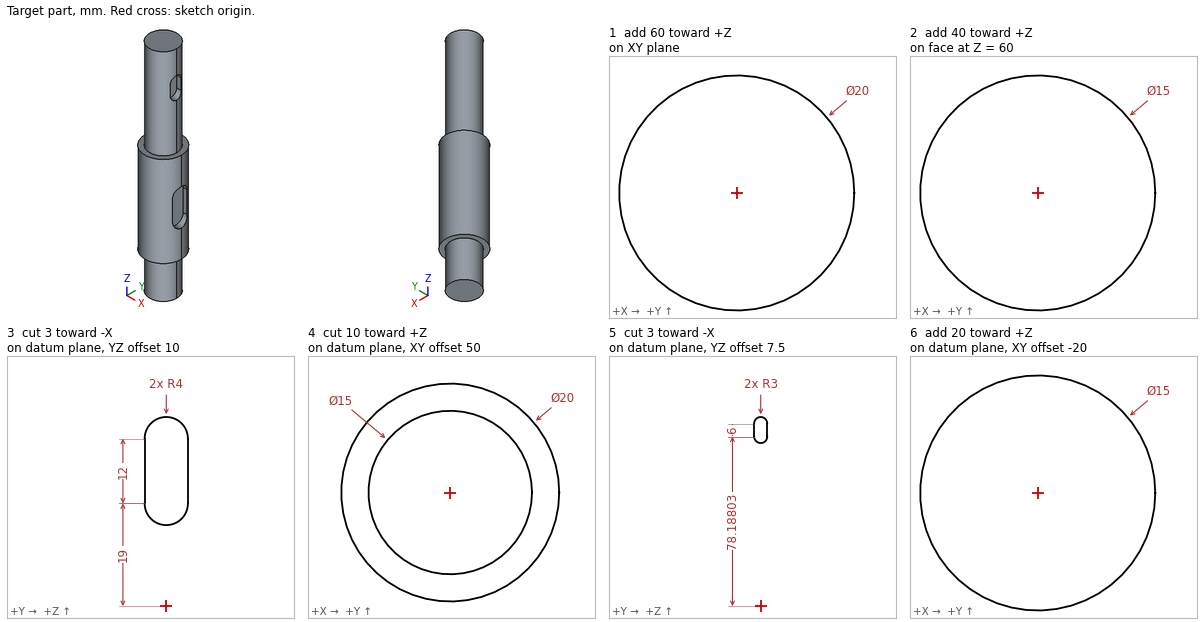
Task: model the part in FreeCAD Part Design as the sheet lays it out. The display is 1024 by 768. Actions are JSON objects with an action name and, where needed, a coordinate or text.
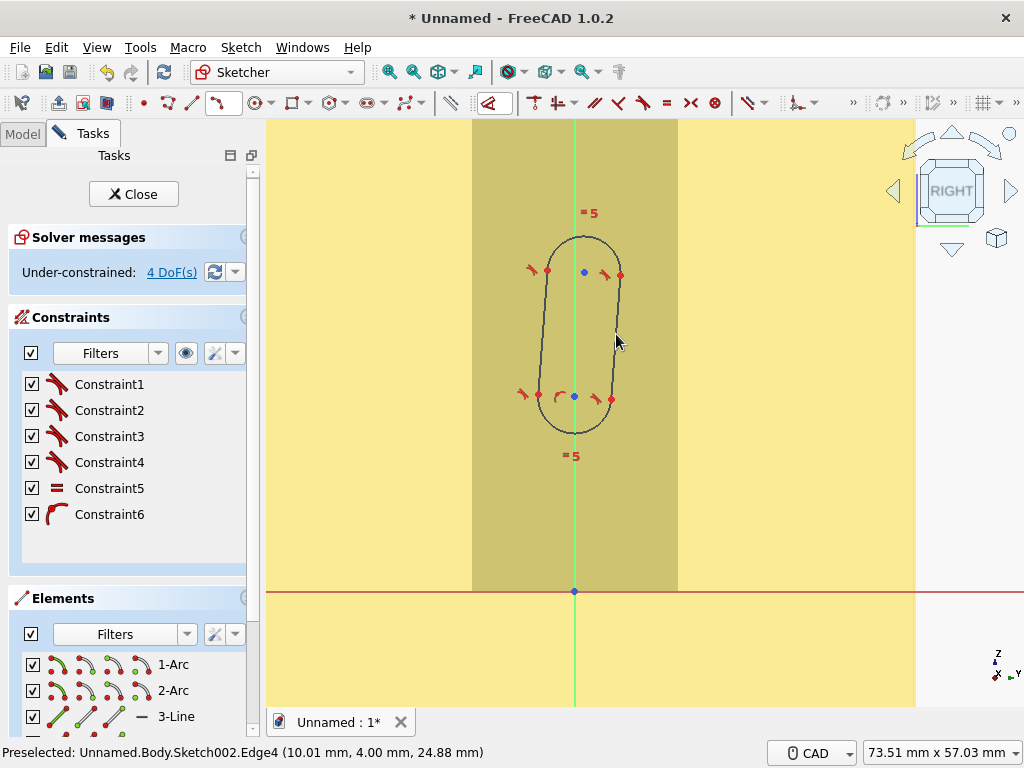
{"action": "left_click", "coordinate": [541, 357]}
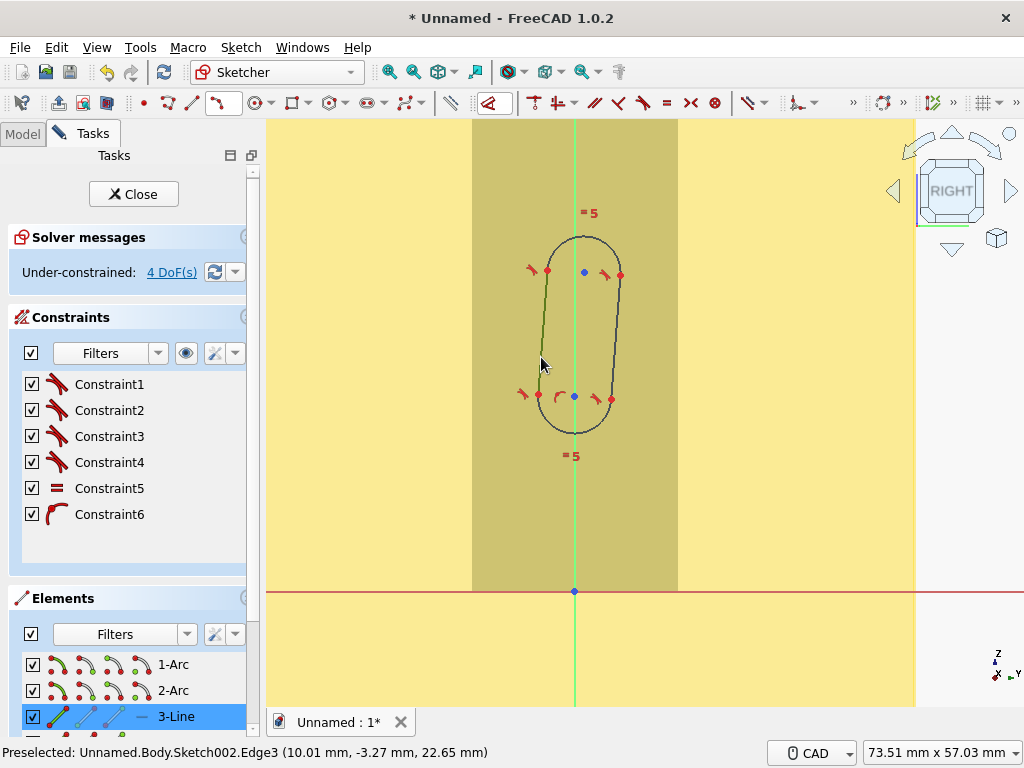
{"action": "left_click", "coordinate": [576, 104]}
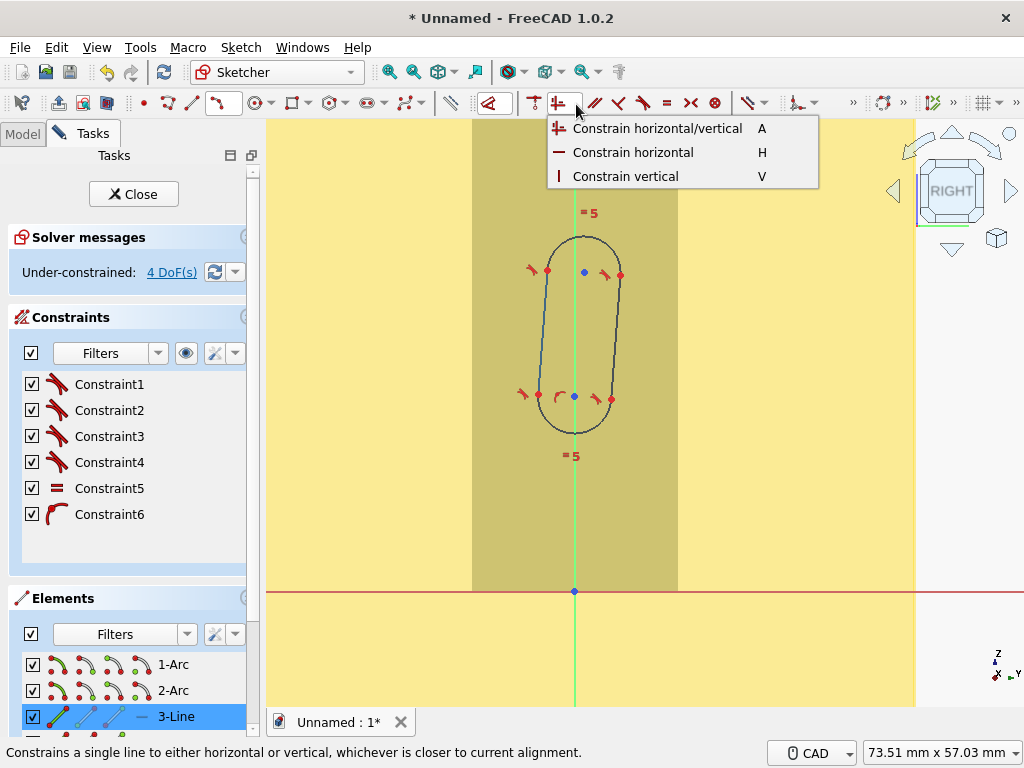
{"action": "left_click", "coordinate": [683, 176]}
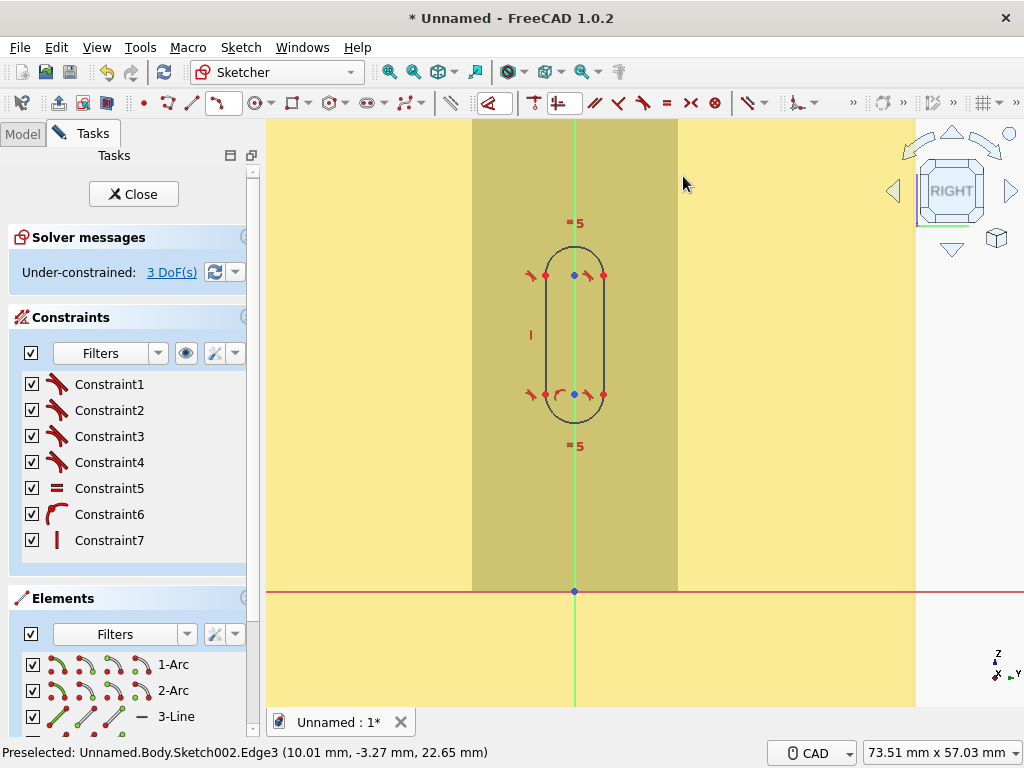
{"action": "left_click", "coordinate": [488, 104]}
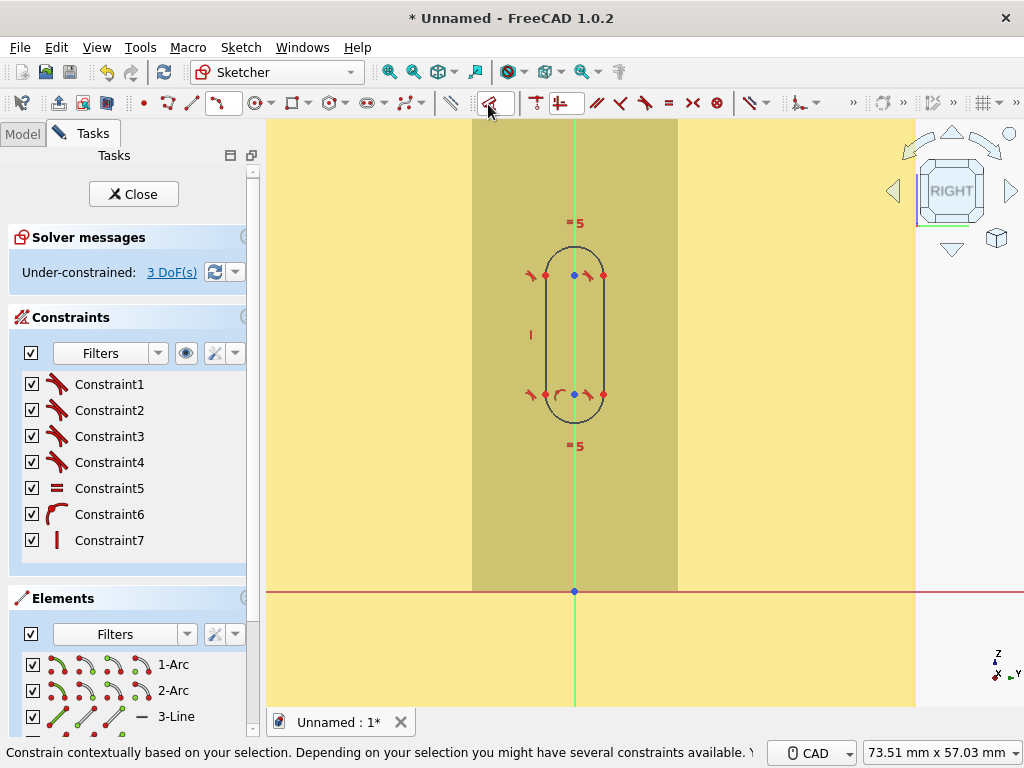
{"action": "left_click", "coordinate": [558, 417]}
{"action": "left_click", "coordinate": [539, 443]}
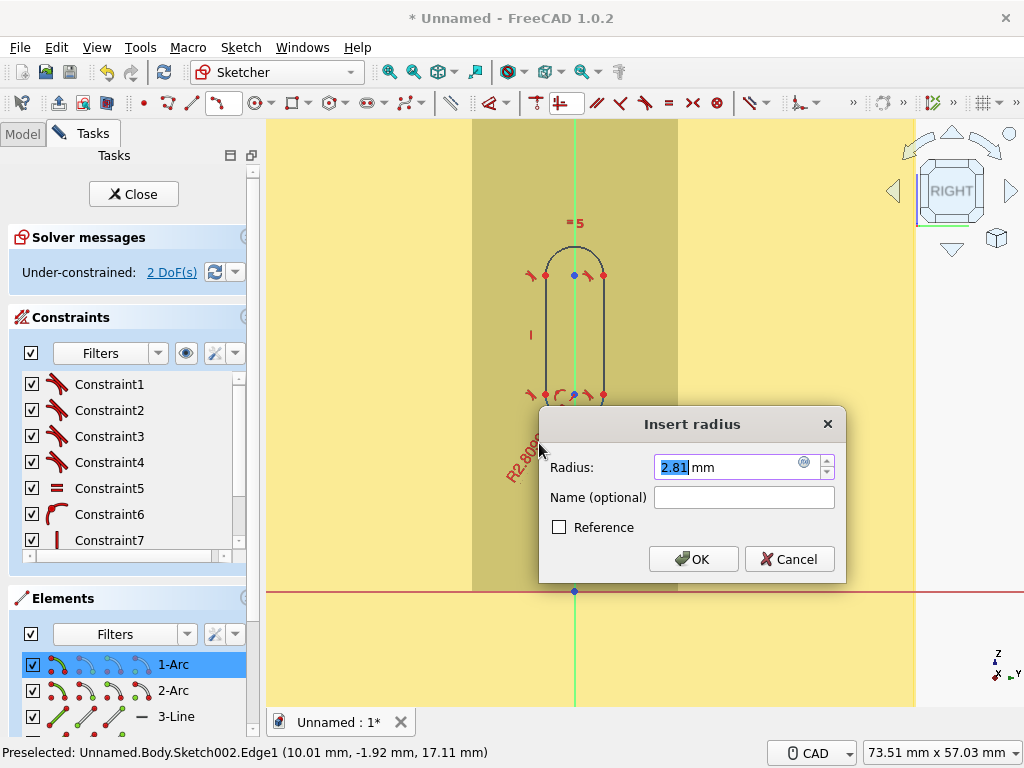
{"action": "type", "text": "4"}
{"action": "key", "text": "Return"}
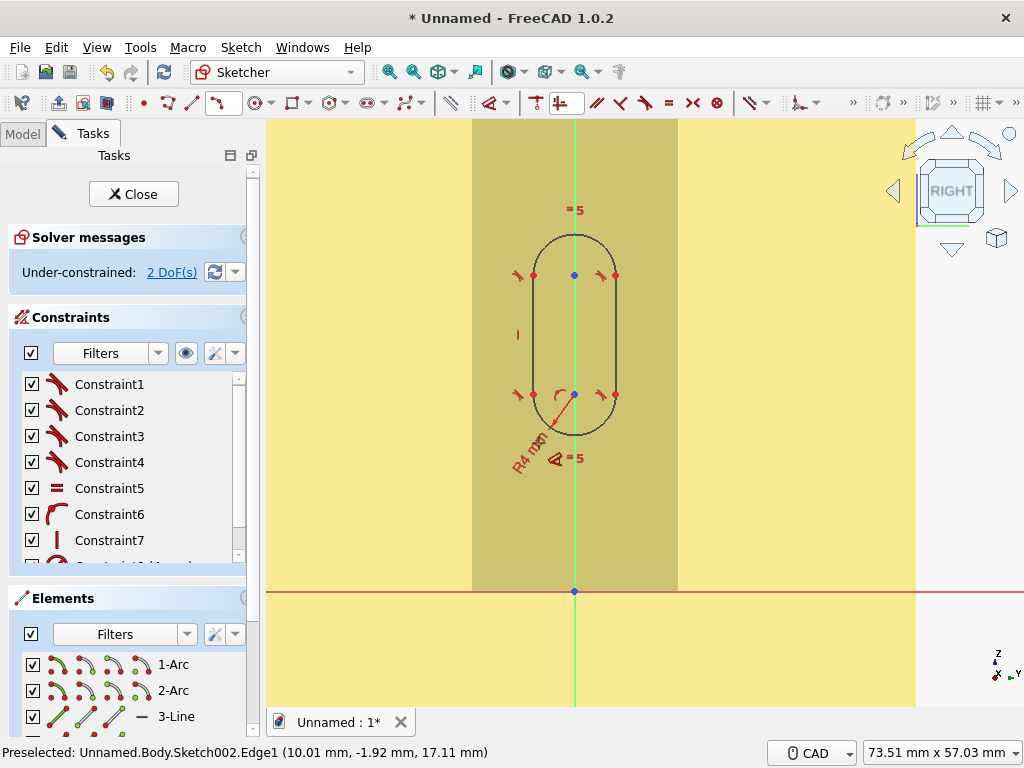
{"action": "left_click", "coordinate": [533, 359]}
{"action": "left_click", "coordinate": [499, 335]}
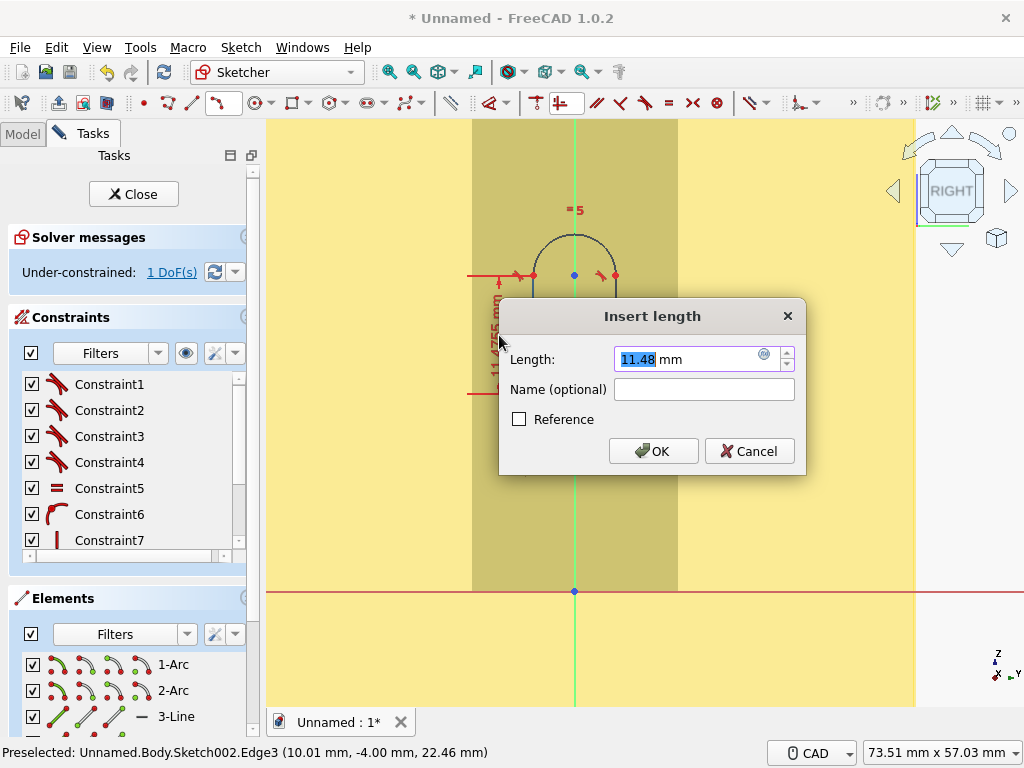
{"action": "type", "text": "12"}
{"action": "key", "text": "Return"}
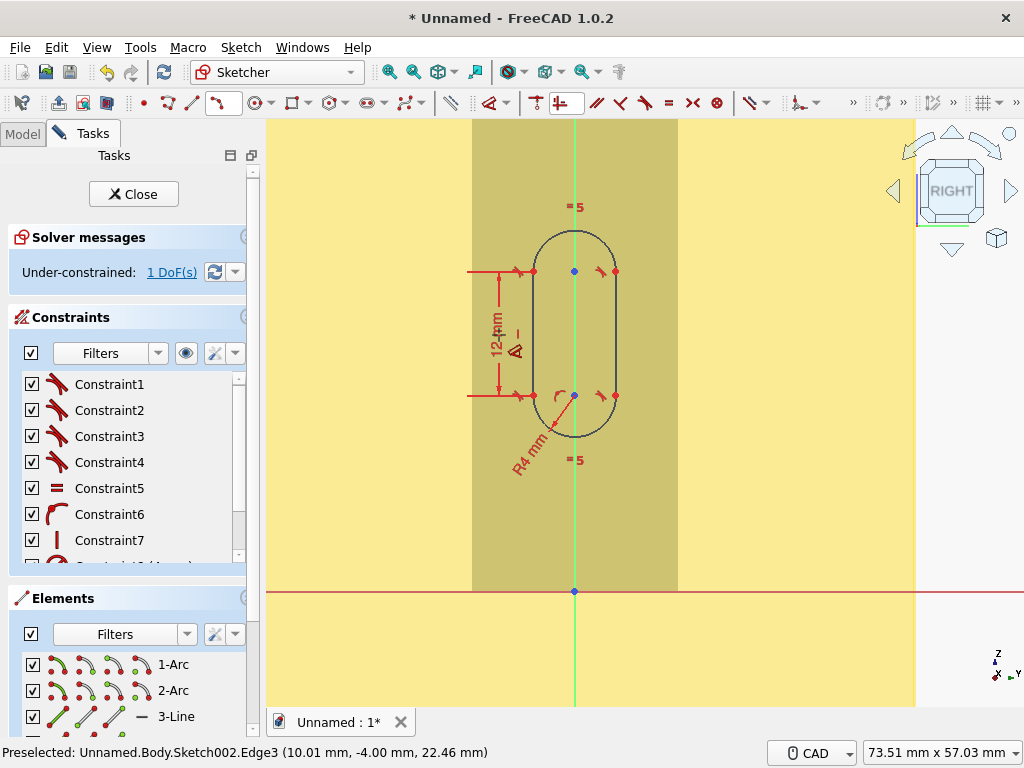
{"action": "left_click", "coordinate": [533, 396]}
{"action": "left_click", "coordinate": [499, 494]}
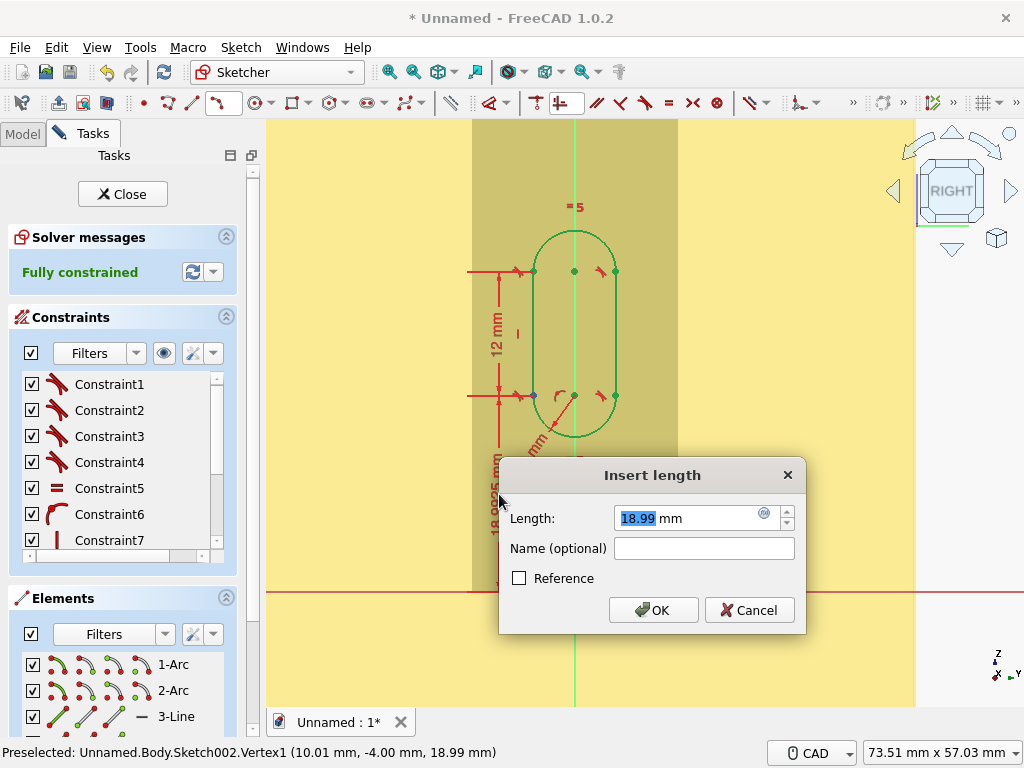
{"action": "type", "text": "19"}
{"action": "key", "text": "Return"}
{"action": "key", "text": "Escape"}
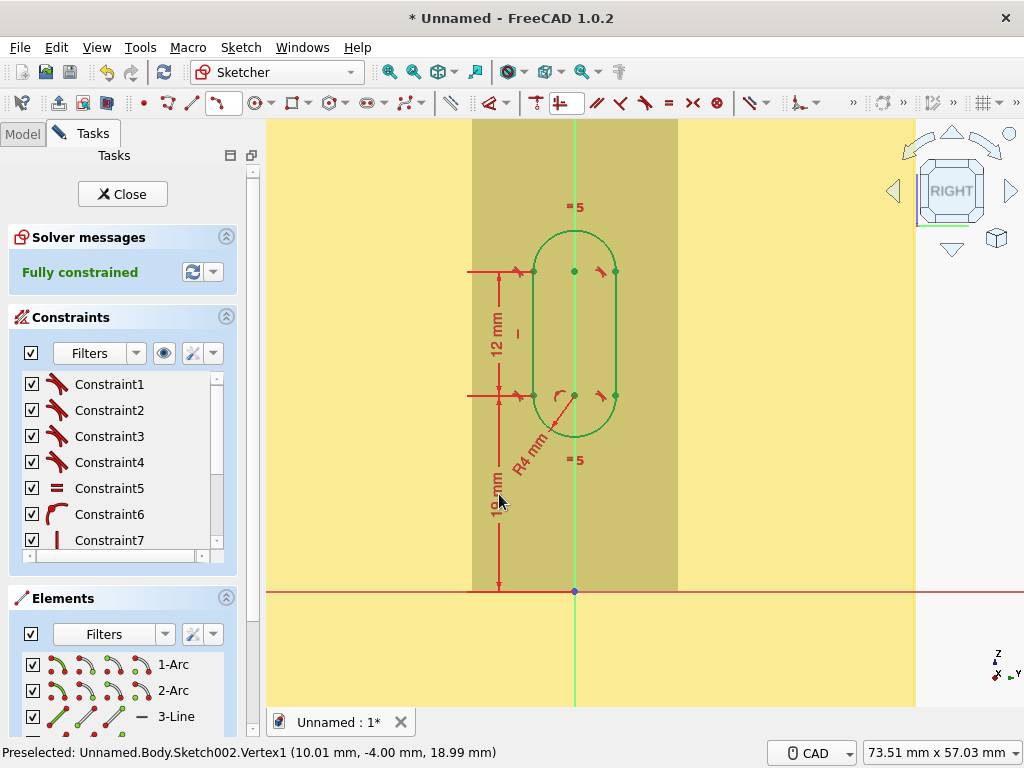
{"action": "left_click", "coordinate": [123, 194]}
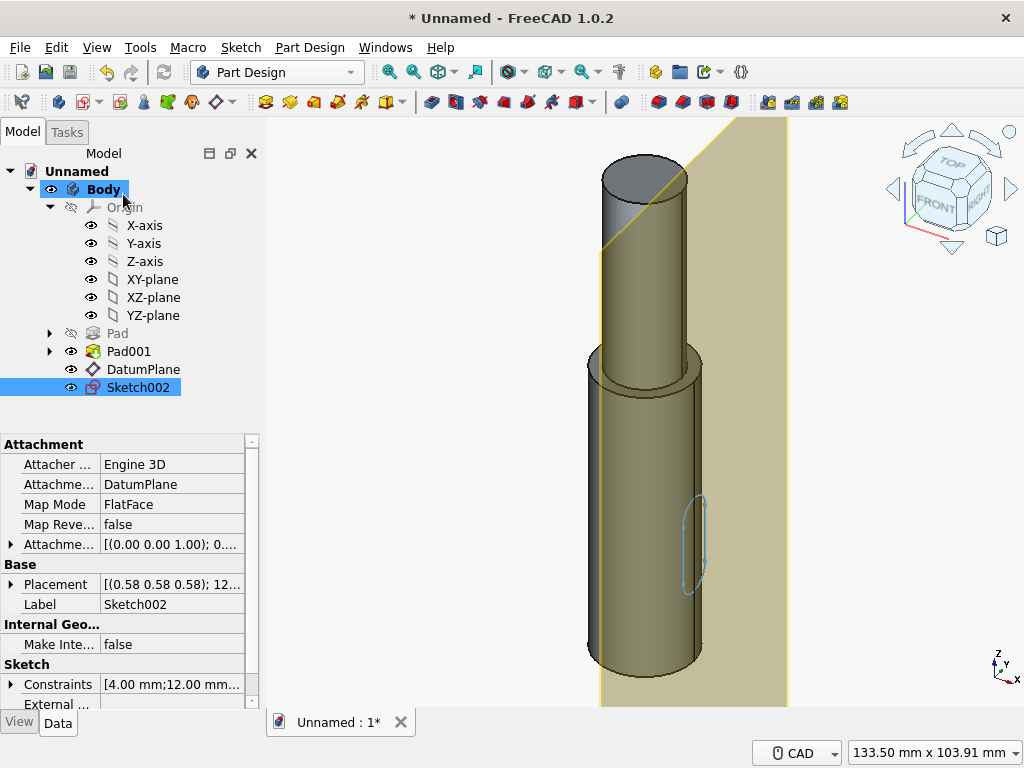
{"action": "left_click", "coordinate": [432, 102]}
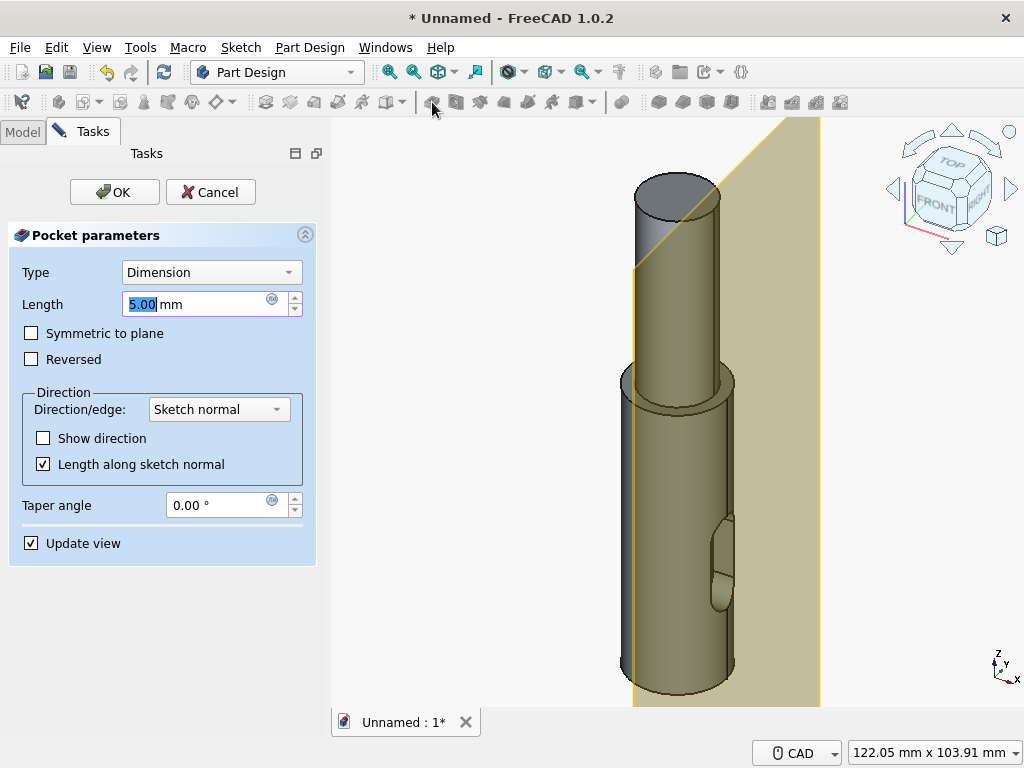
{"action": "type", "text": "3"}
{"action": "key", "text": "Tab"}